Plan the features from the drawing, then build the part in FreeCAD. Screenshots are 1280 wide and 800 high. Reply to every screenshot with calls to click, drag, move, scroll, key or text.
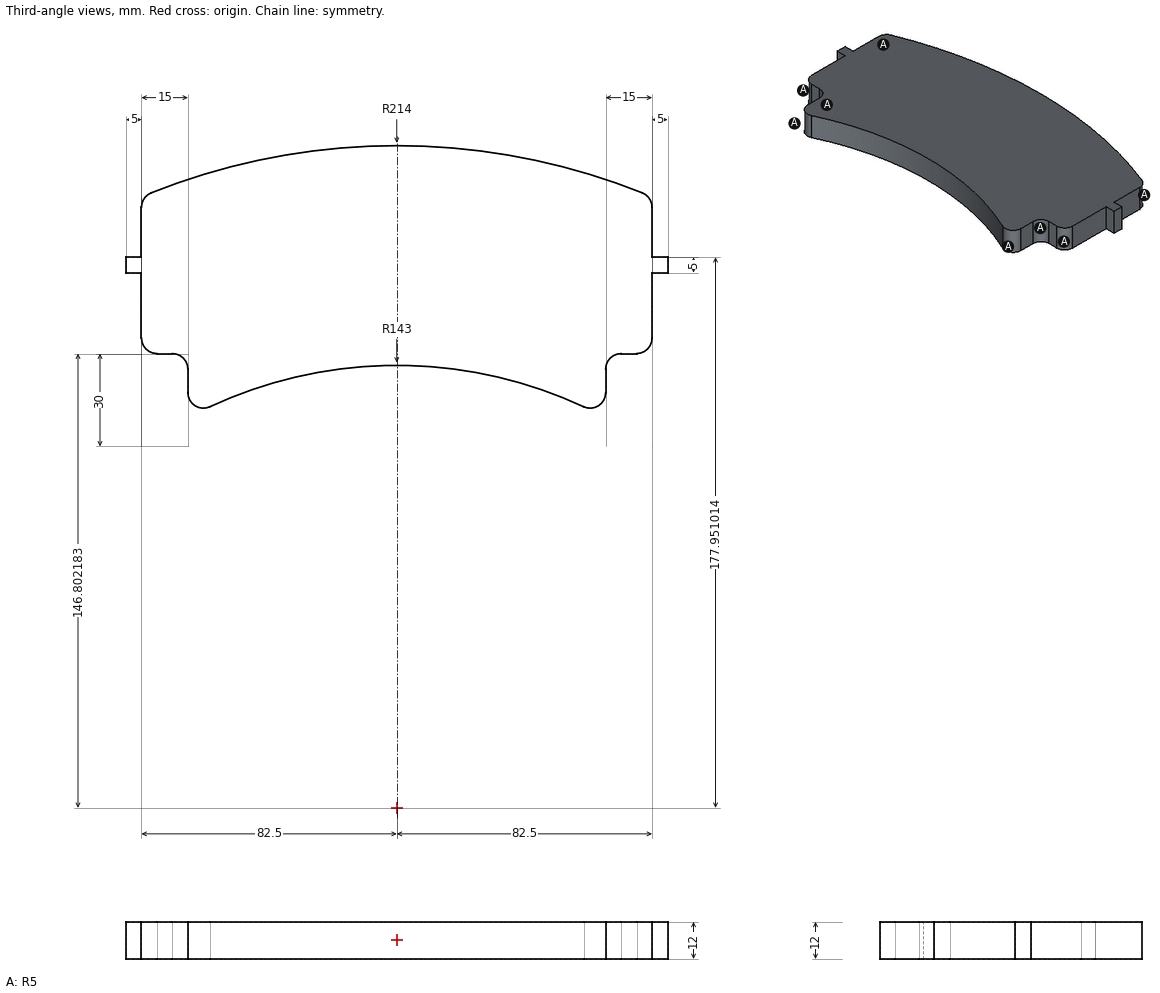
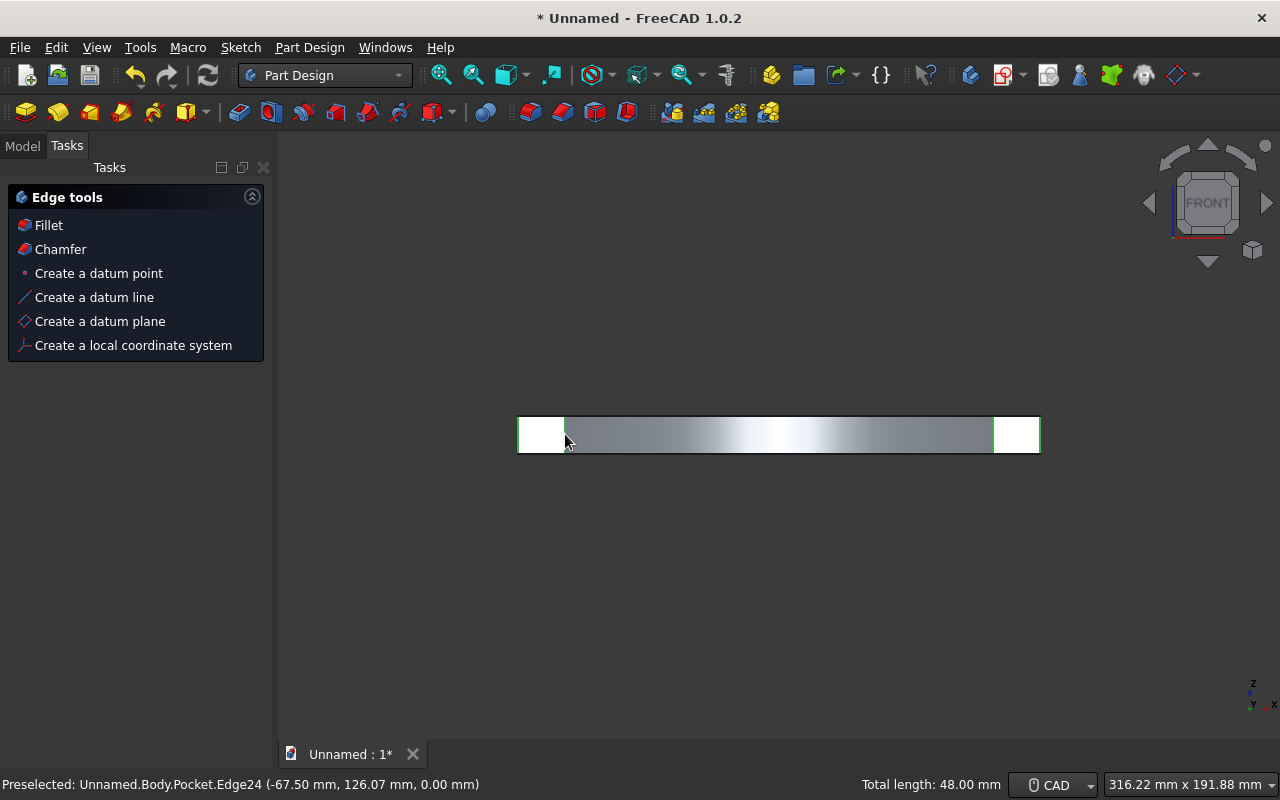
key(3)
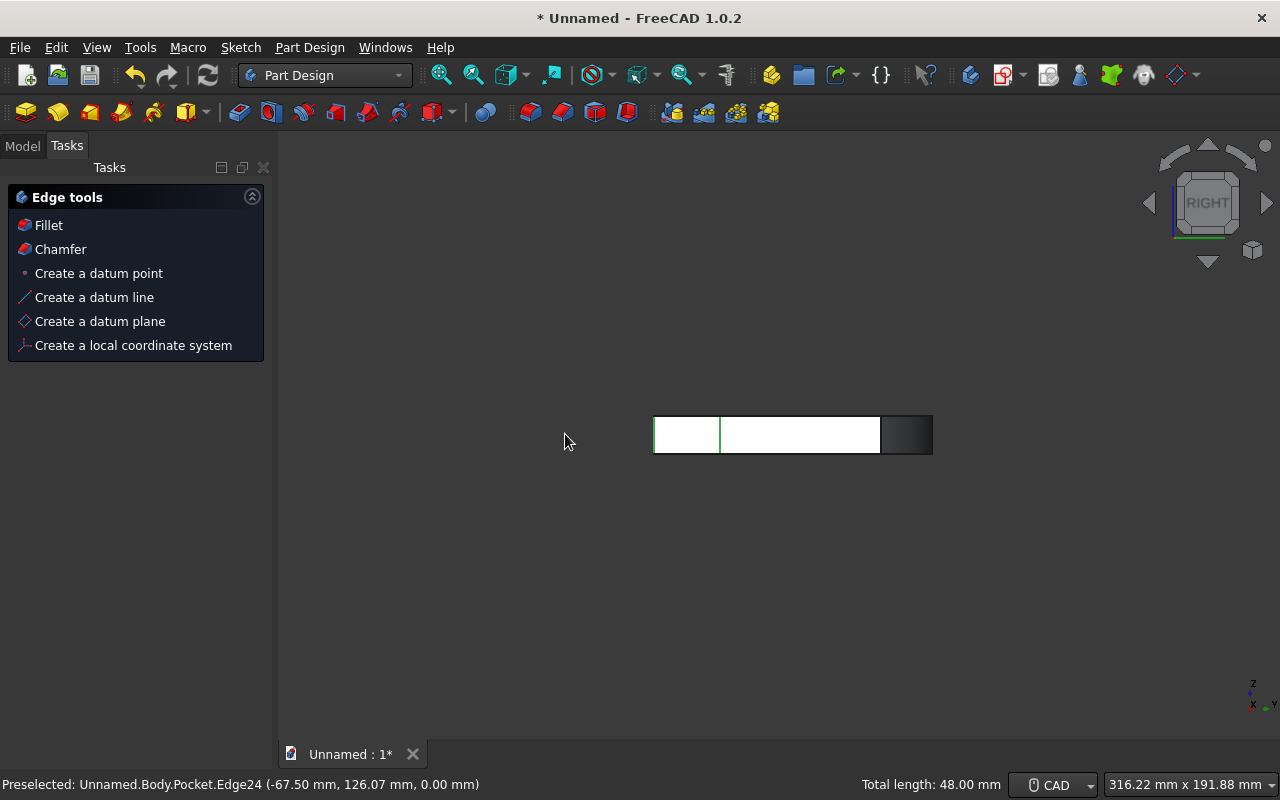
click(442, 76)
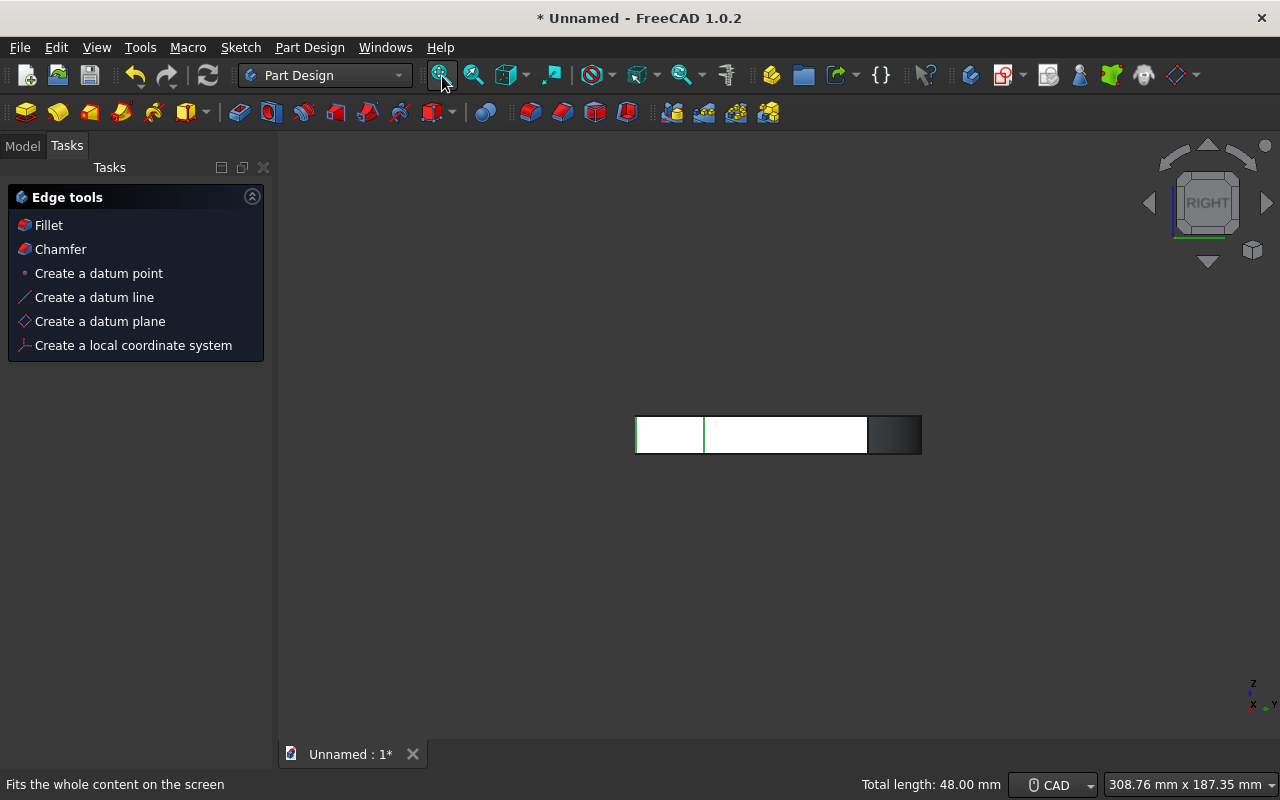
click(868, 434, ctrl)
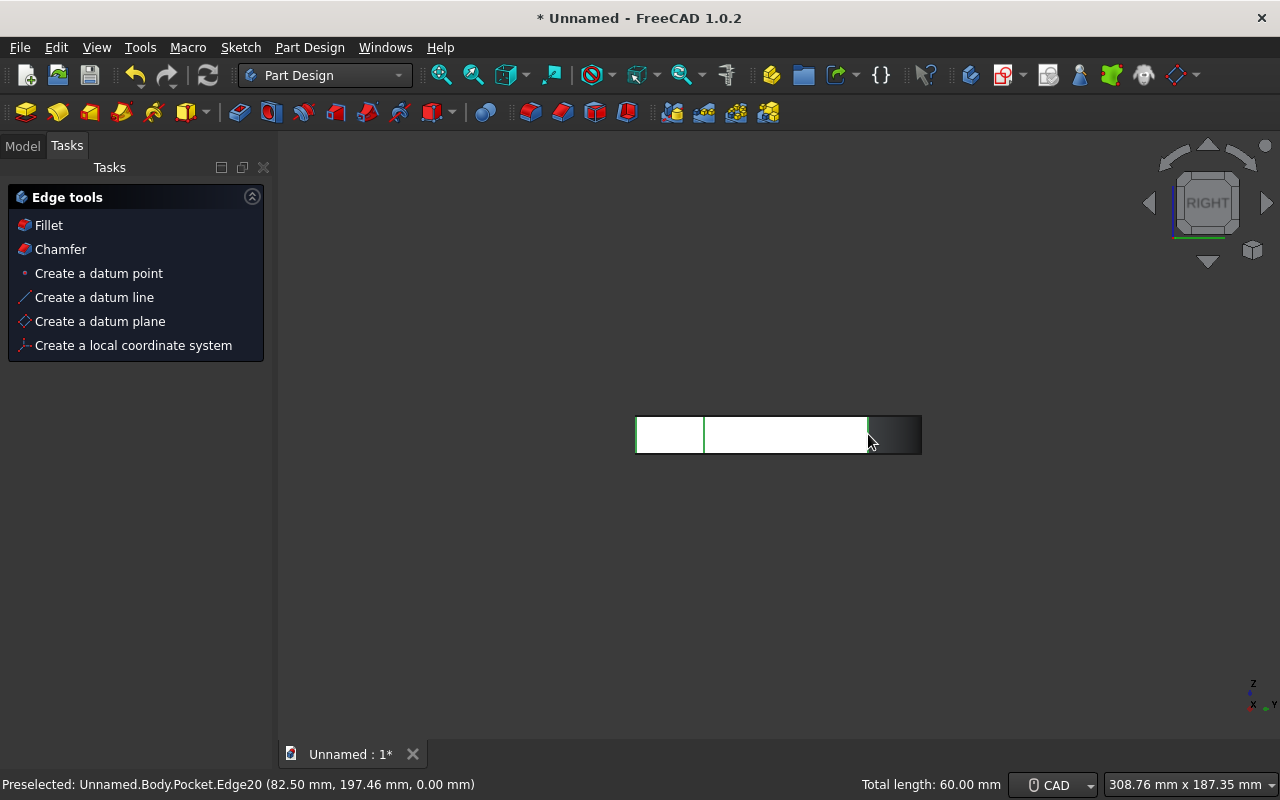
key(5)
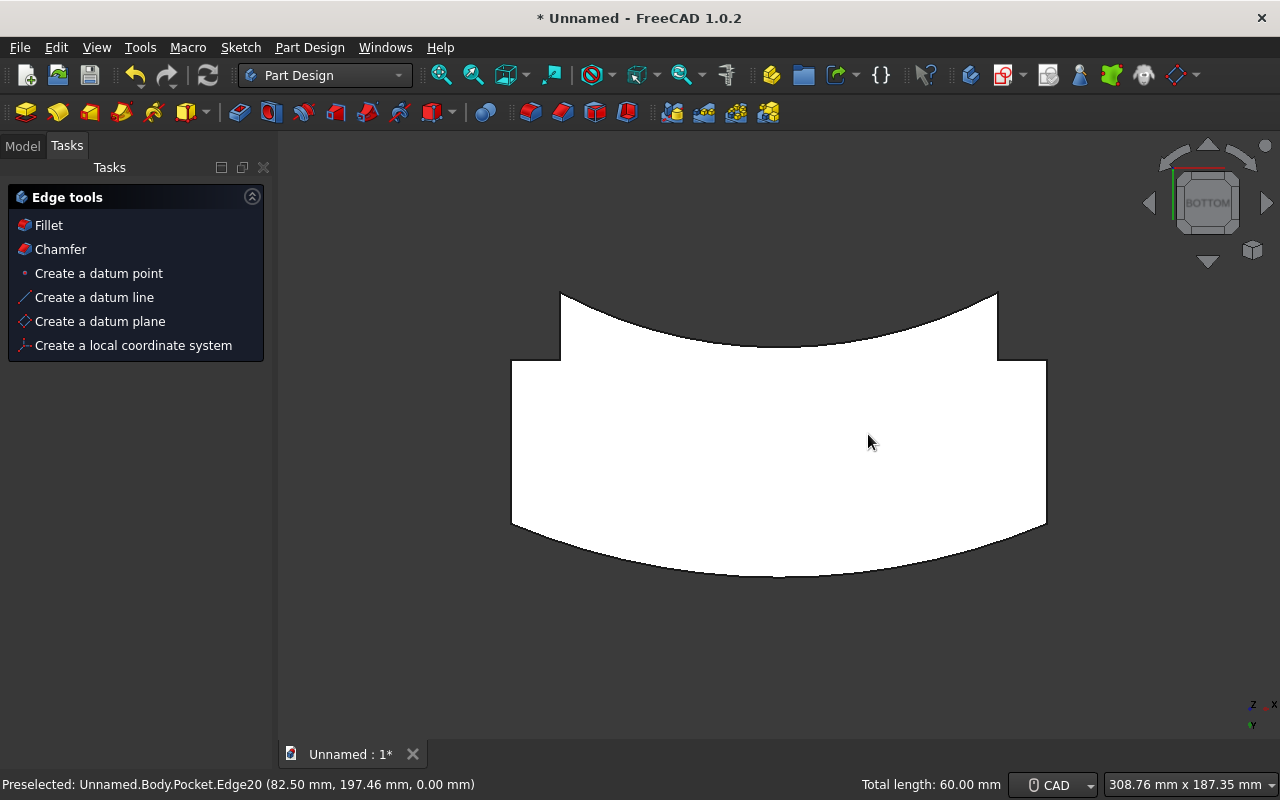
key(4)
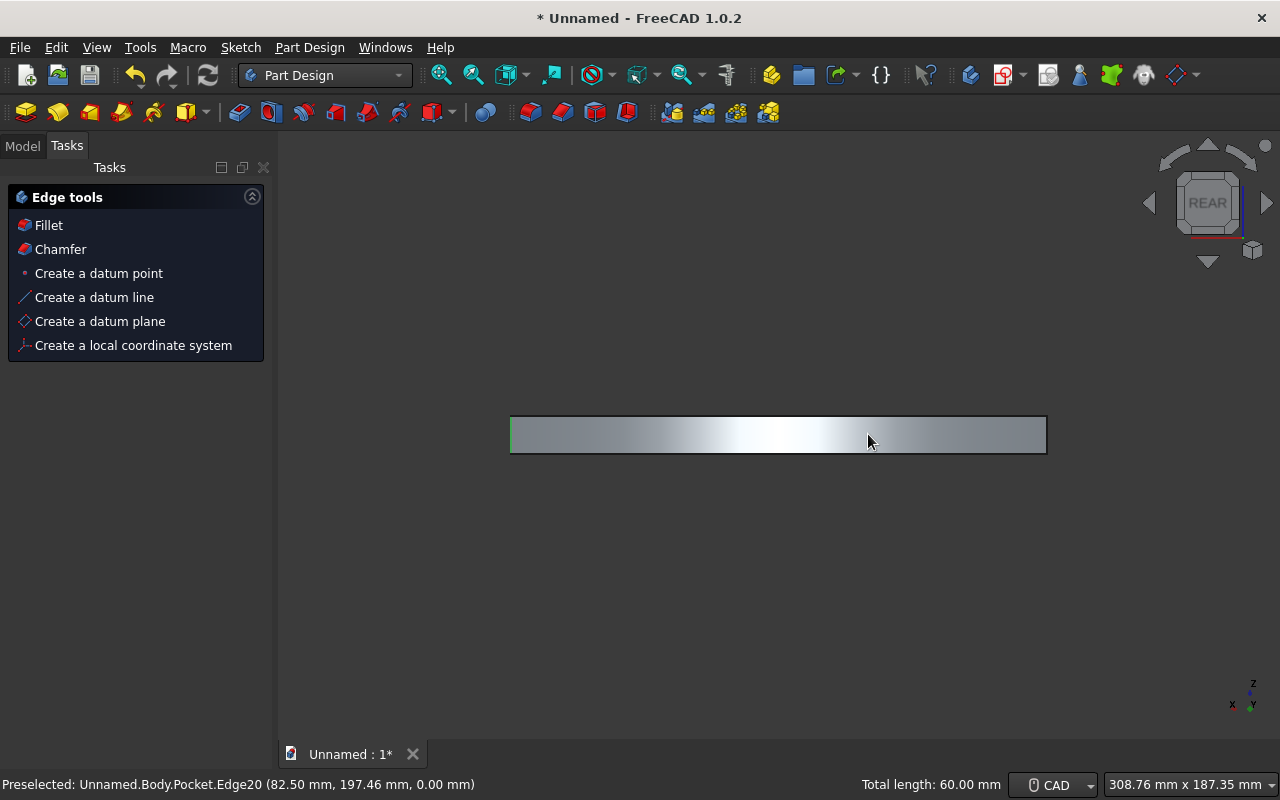
key(6)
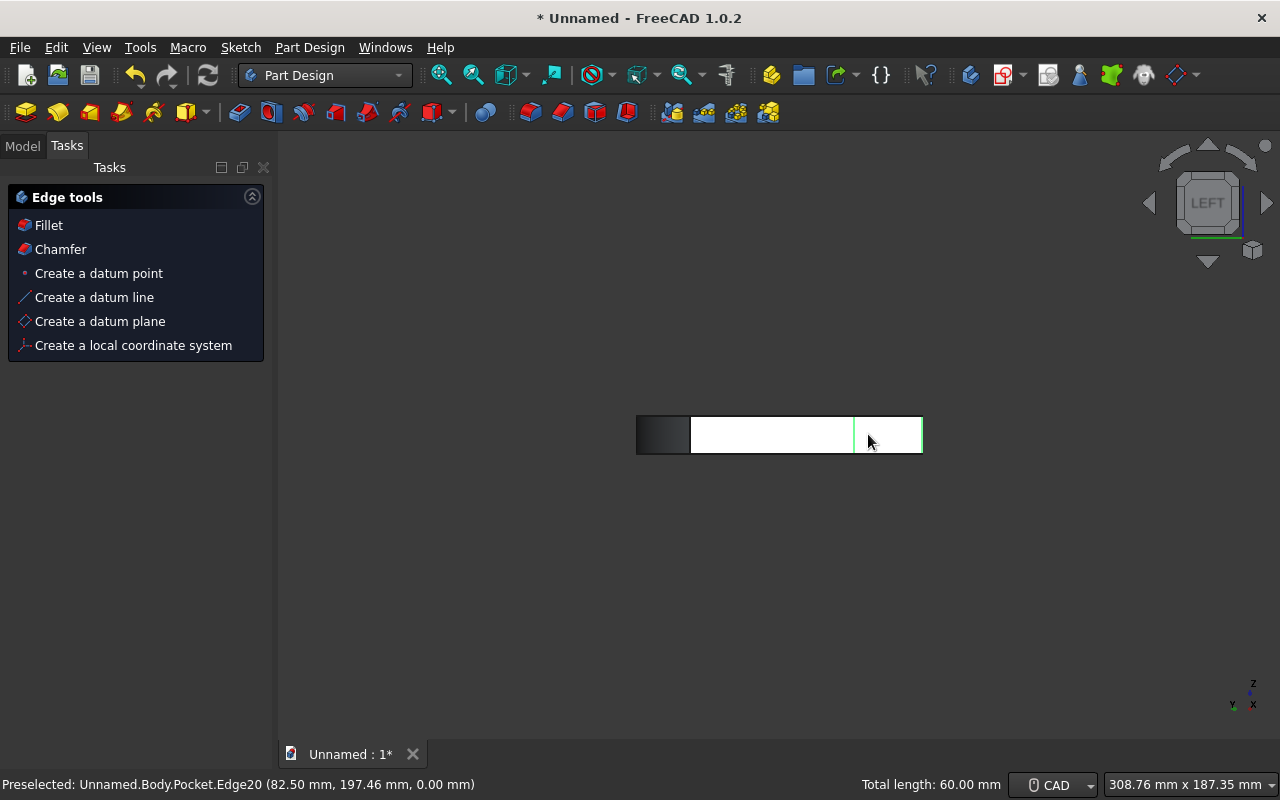
click(442, 76)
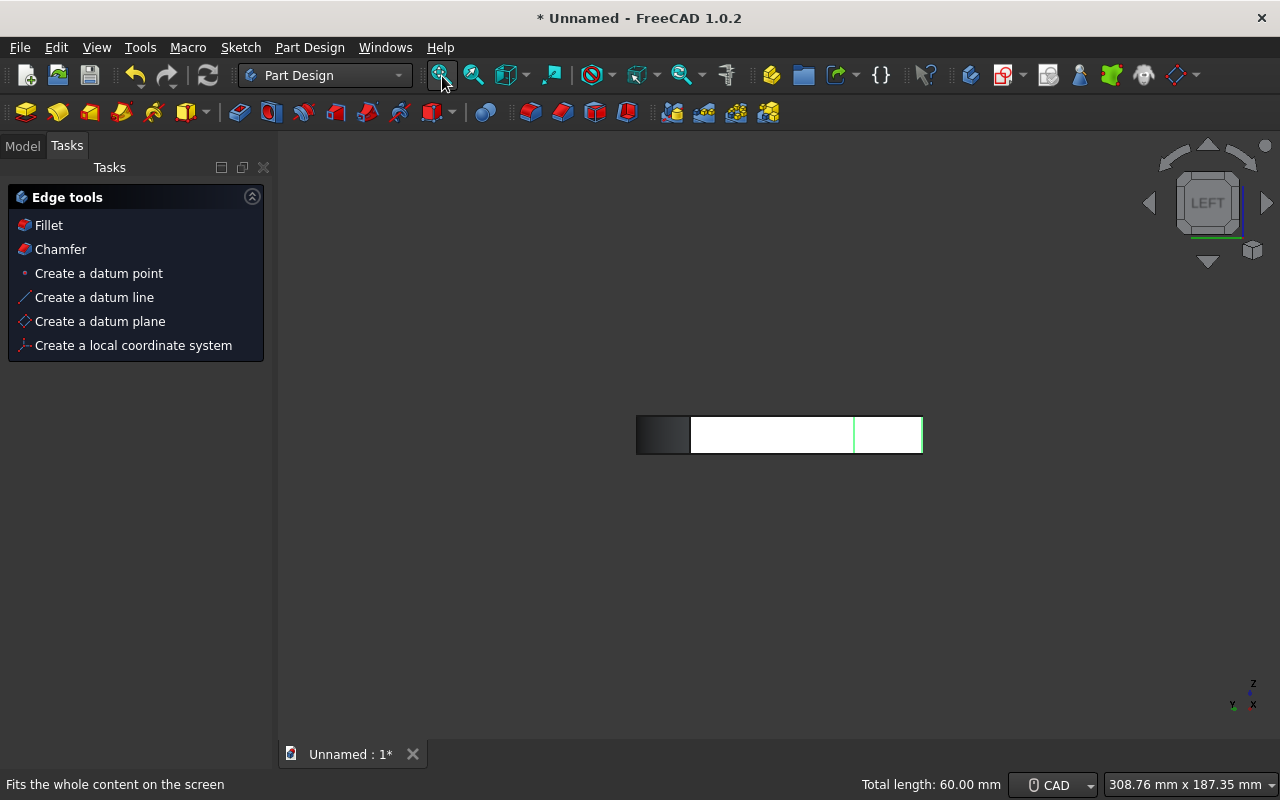
click(690, 434, ctrl)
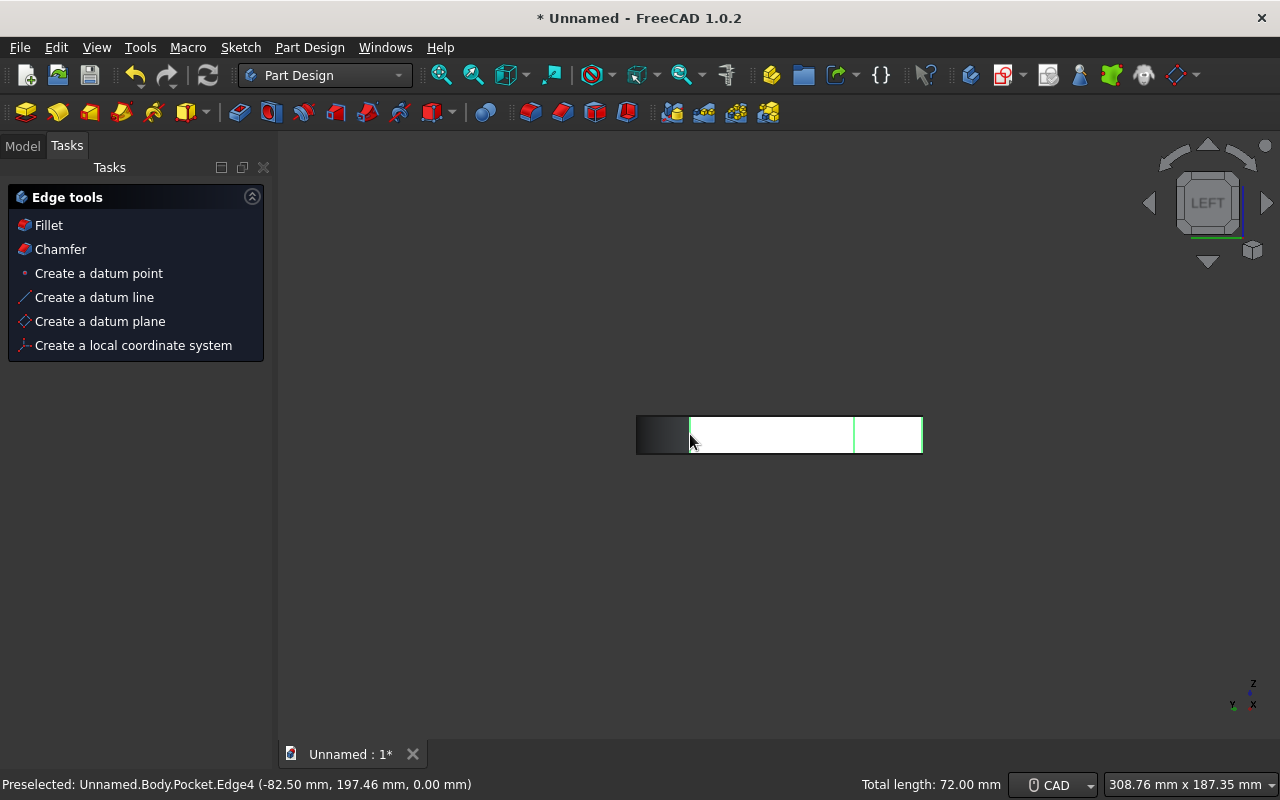
key(v)
key(3)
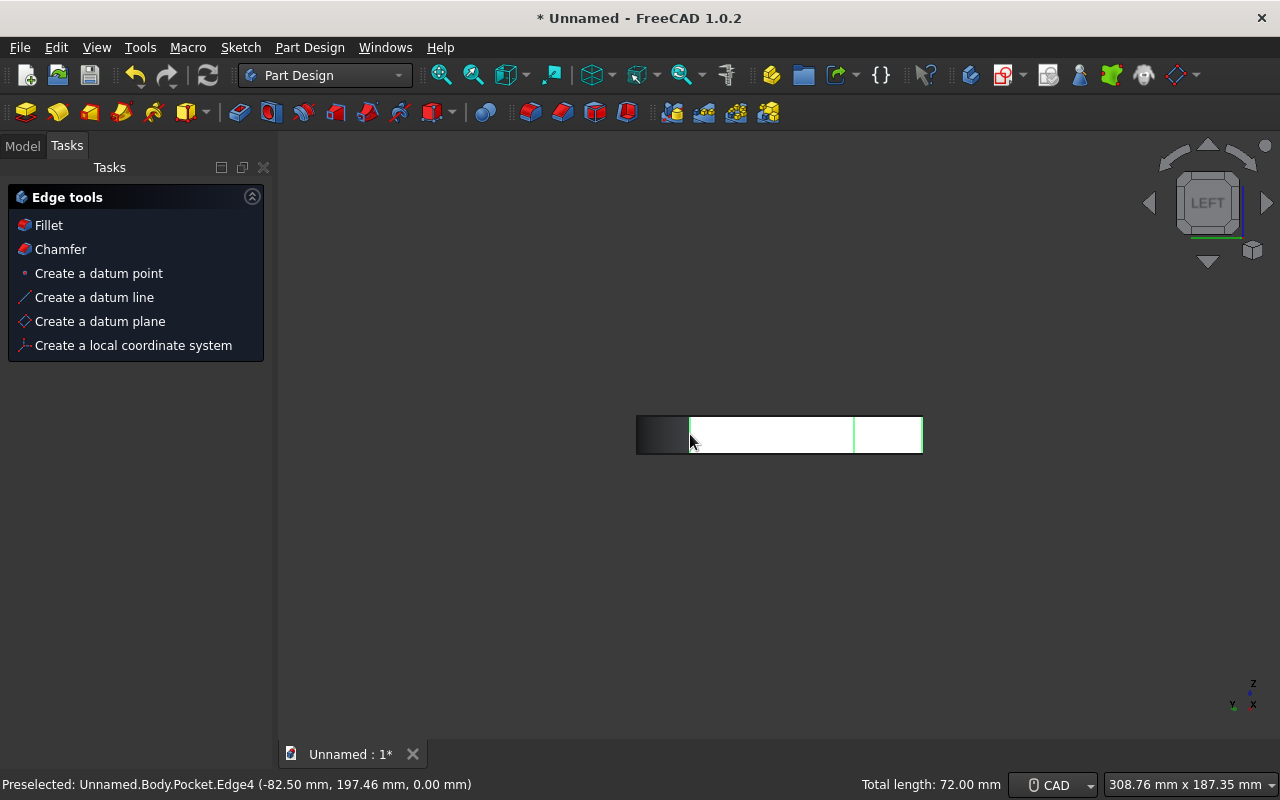
key(0)